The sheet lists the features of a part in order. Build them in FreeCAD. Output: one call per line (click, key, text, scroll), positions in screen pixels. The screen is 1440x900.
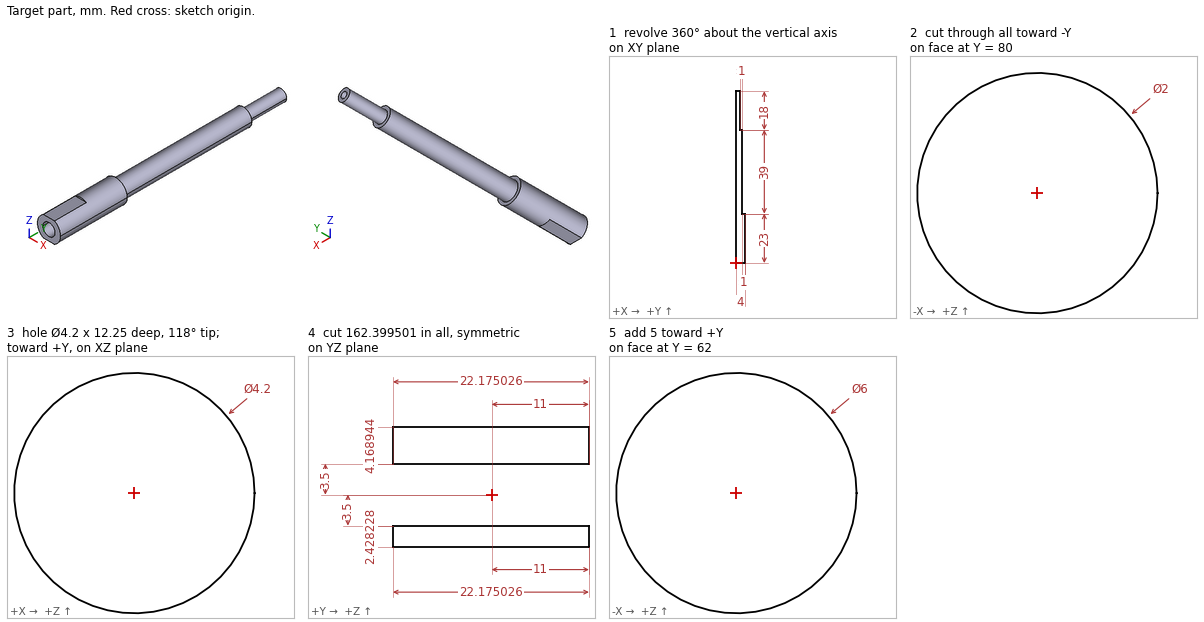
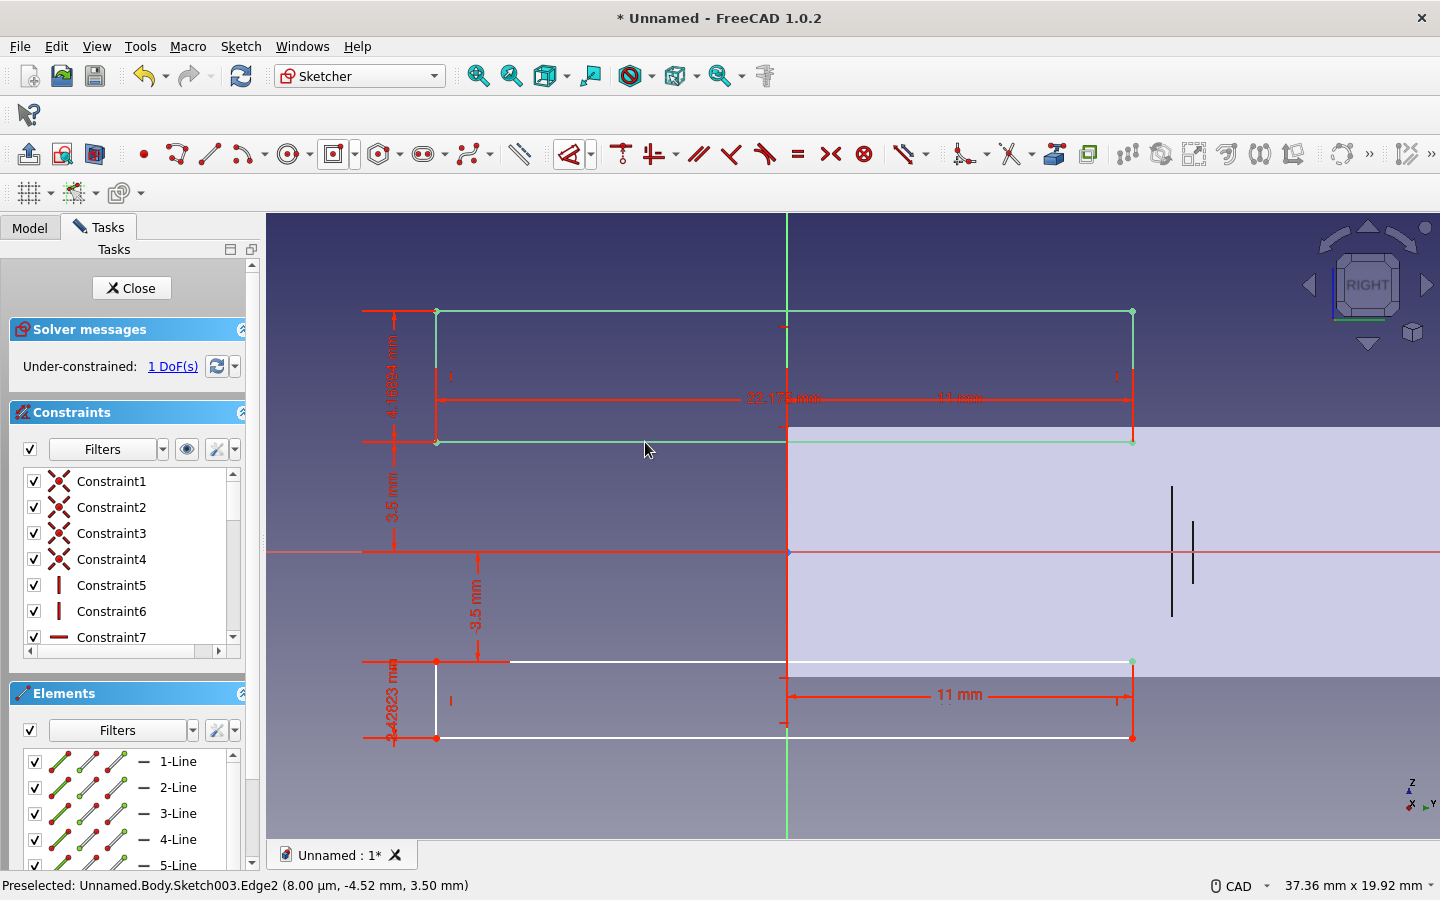
click(645, 738)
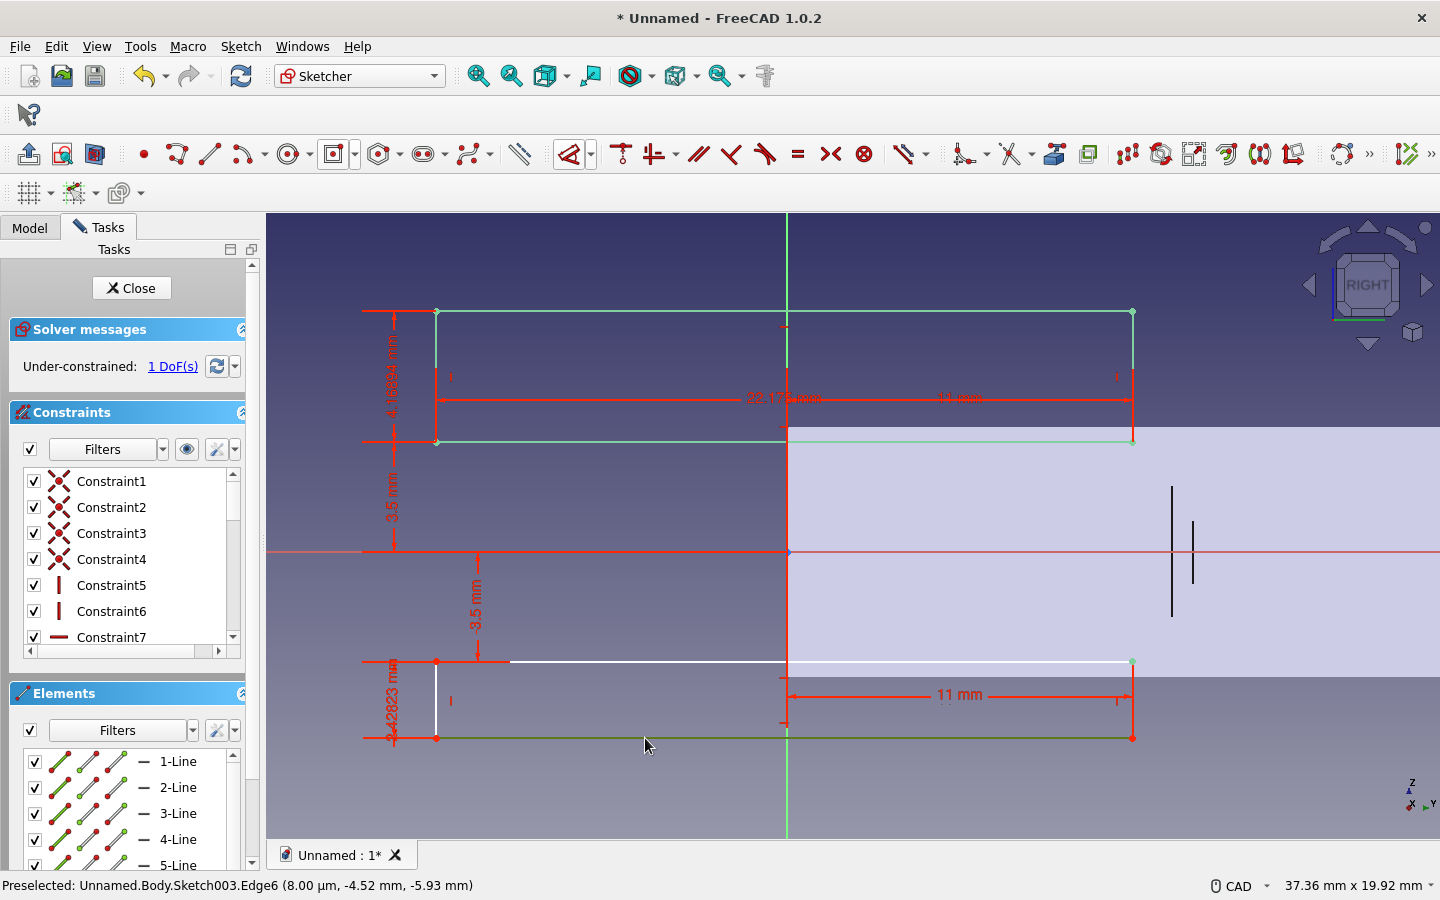
click(590, 154)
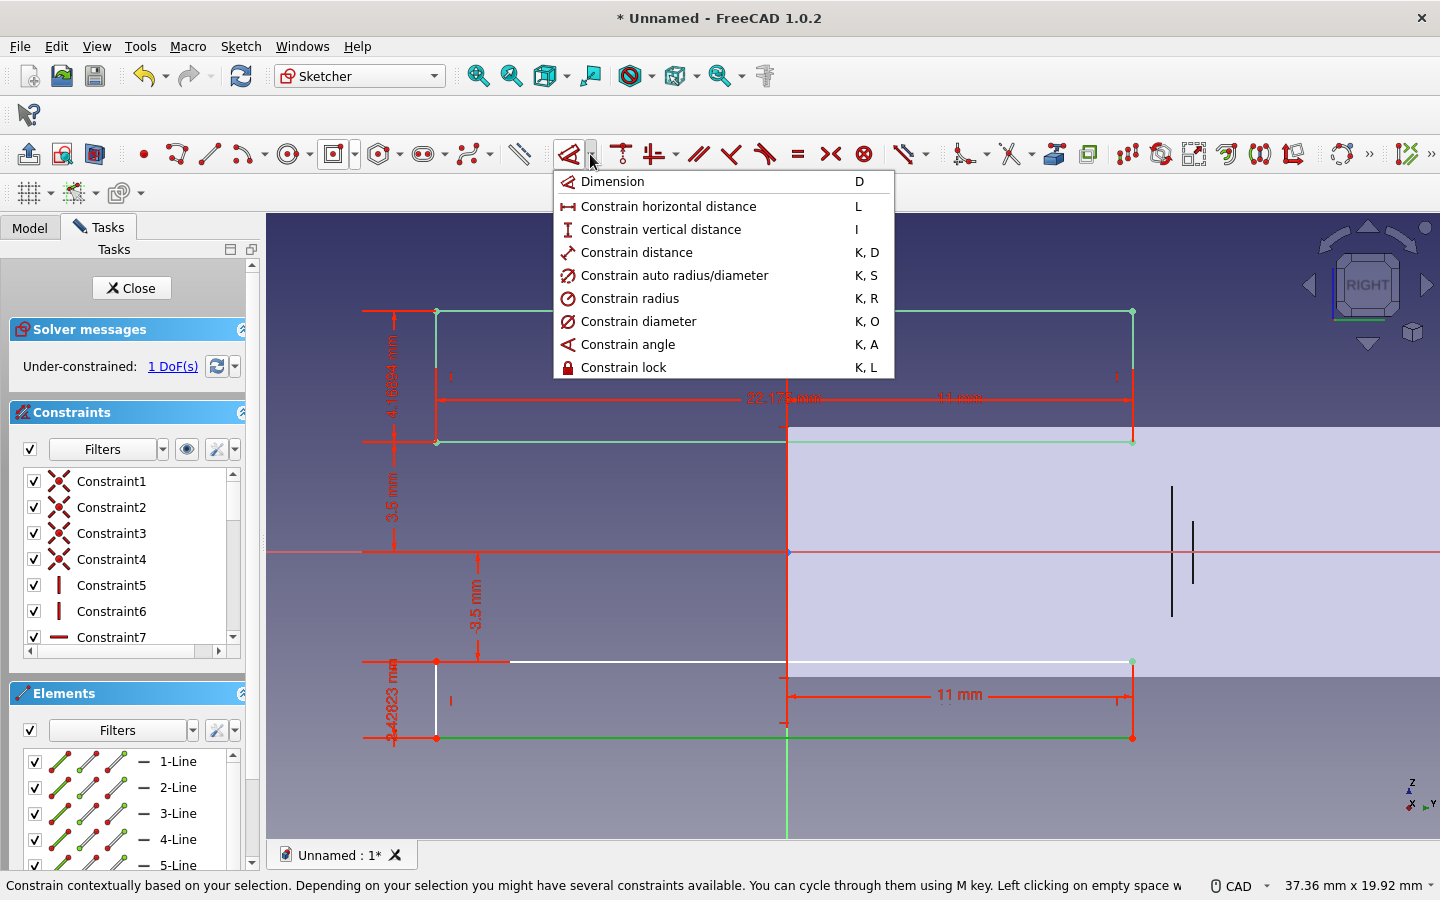
click(724, 206)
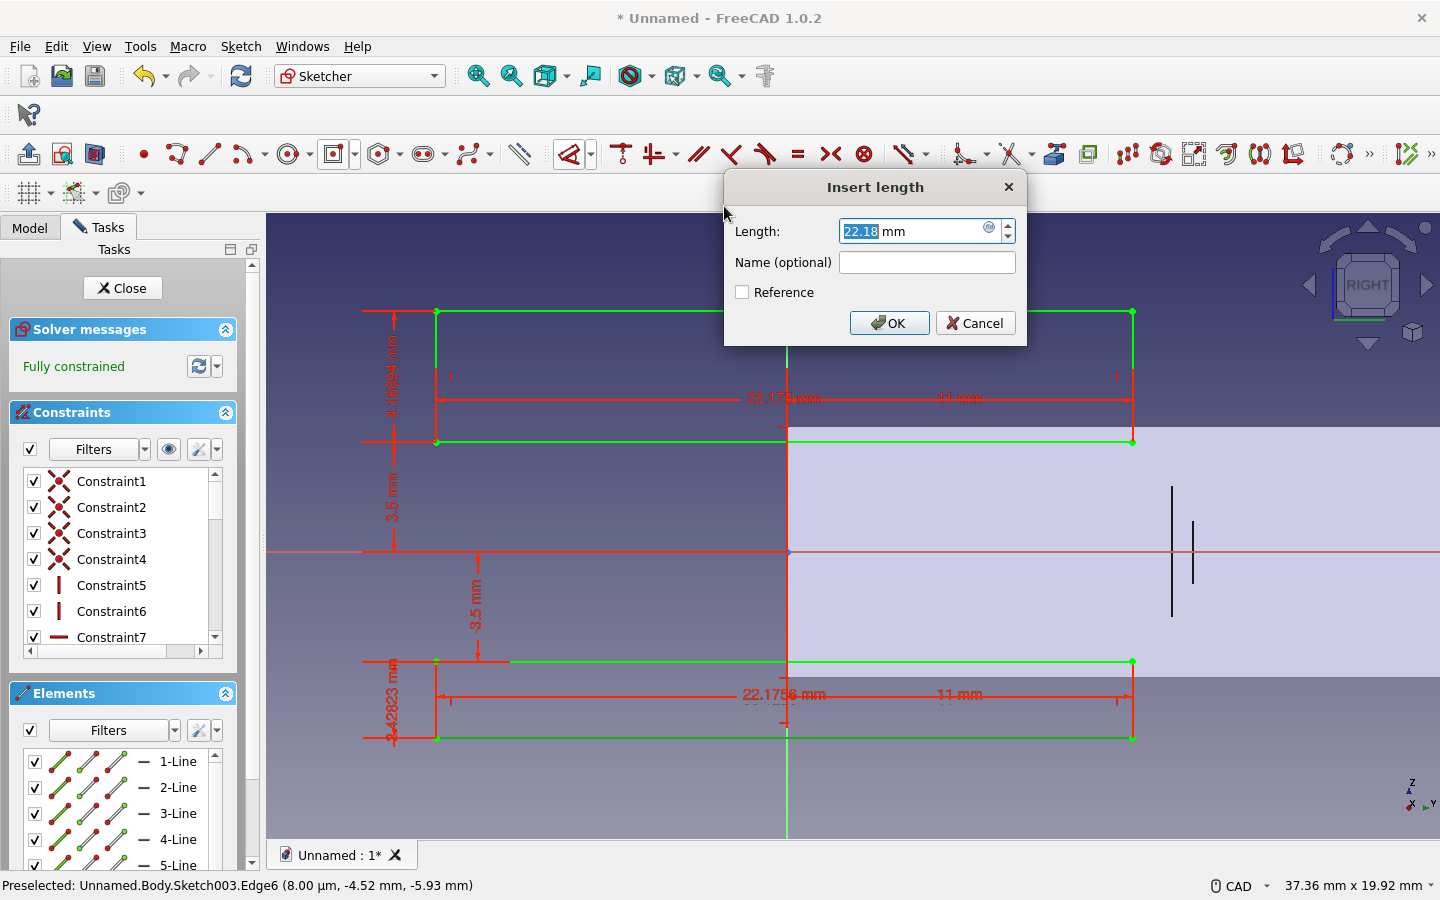
text(22.175026)
key(Return)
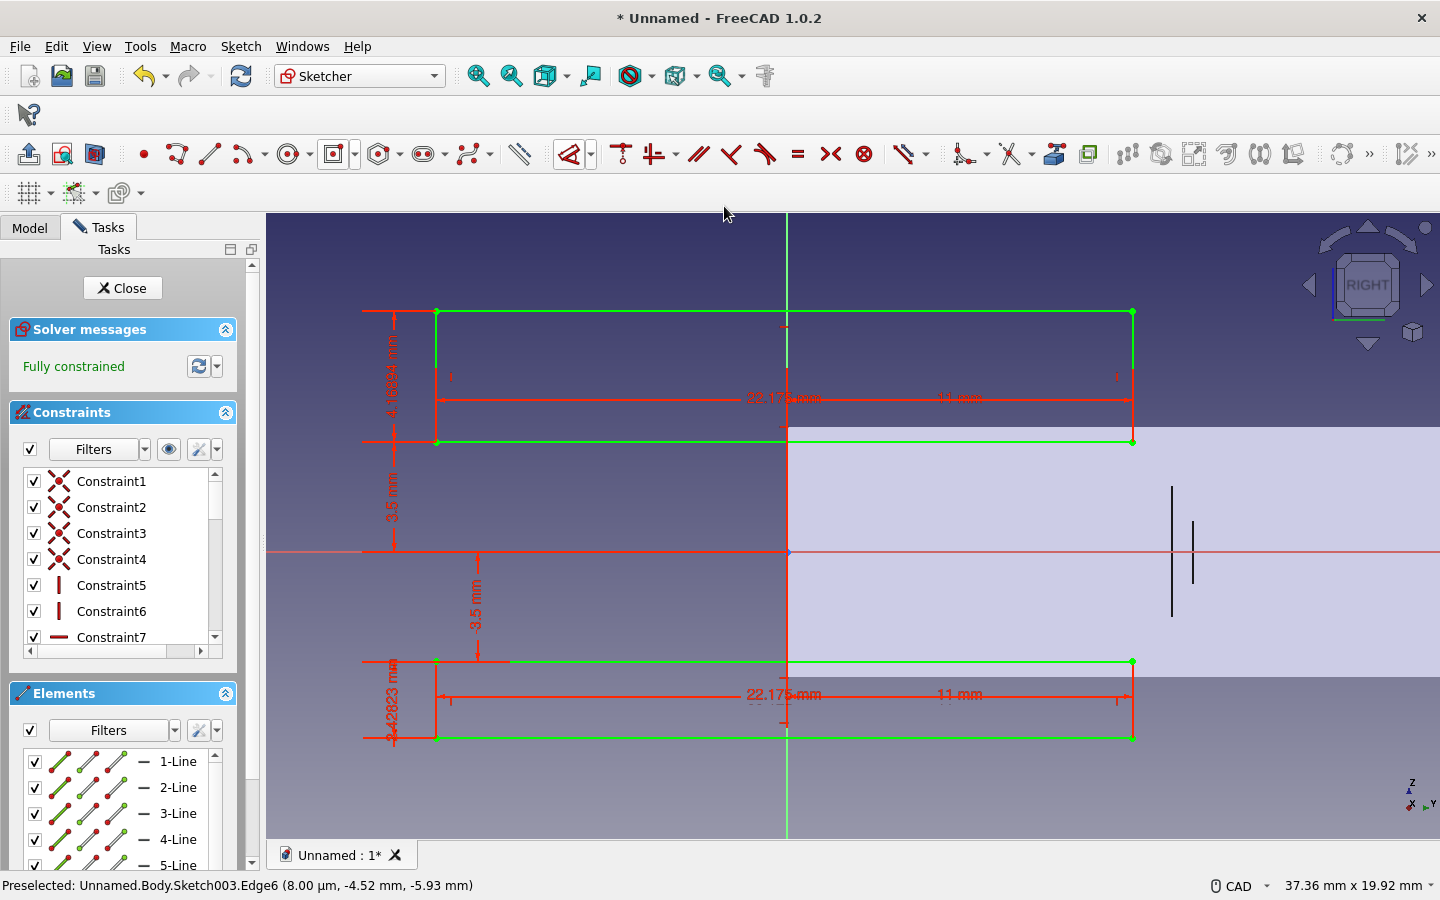
click(123, 288)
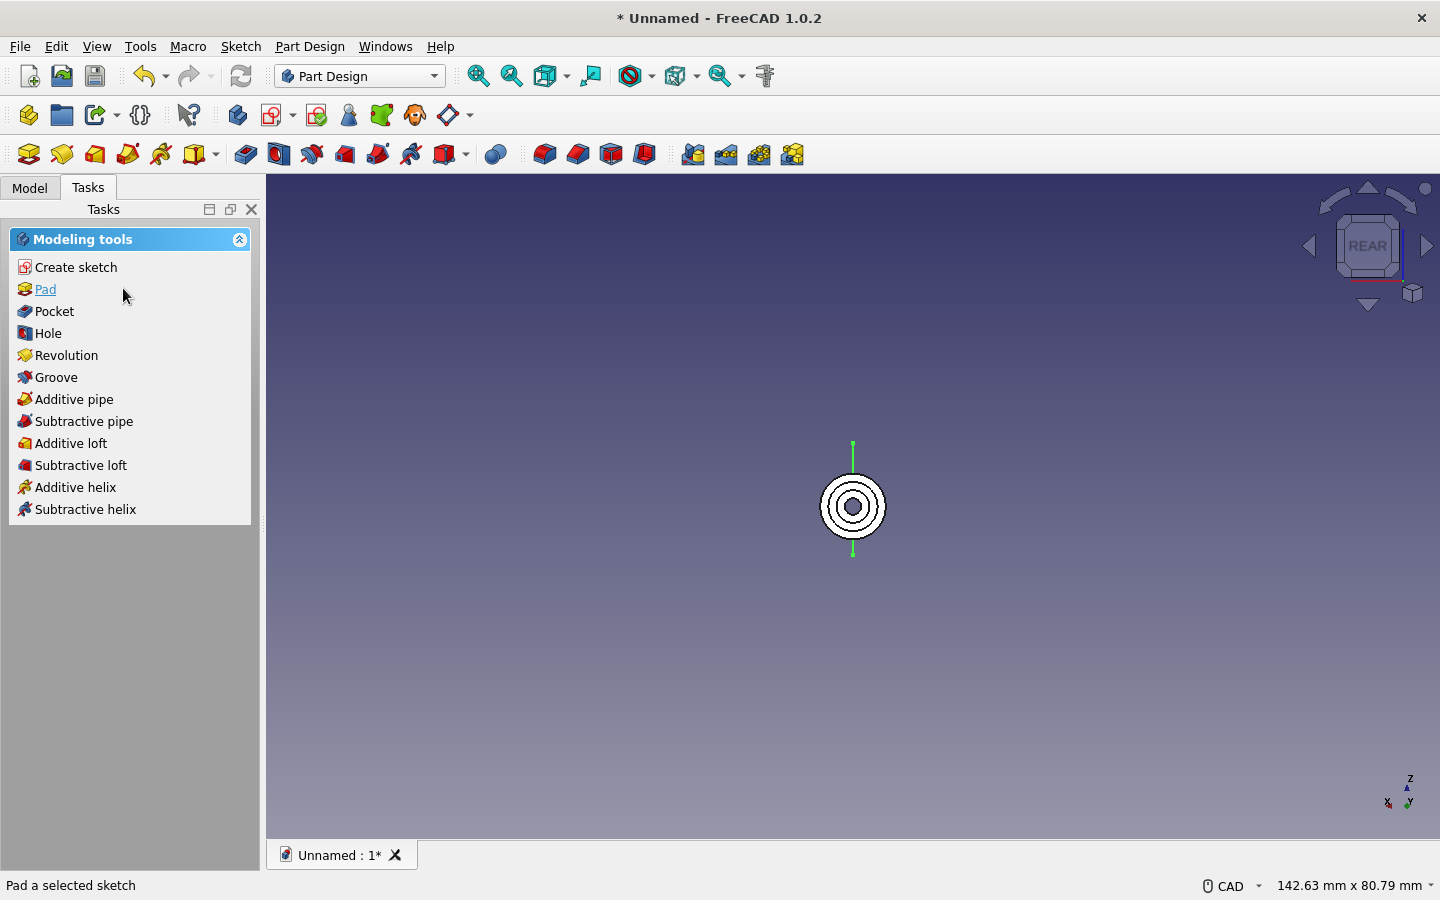
click(246, 154)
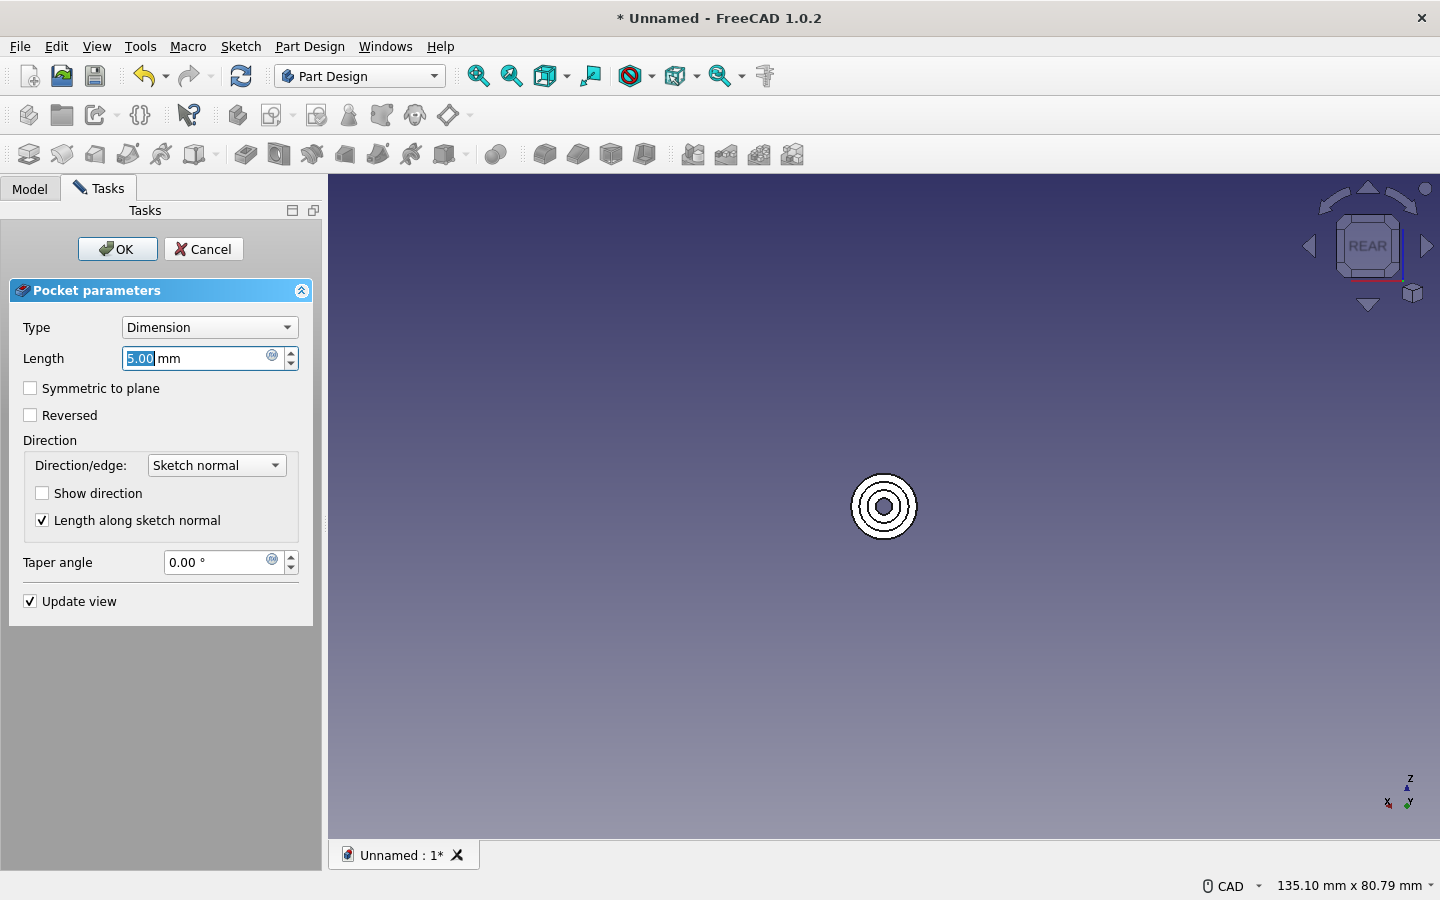
text(162.399501)
key(Tab)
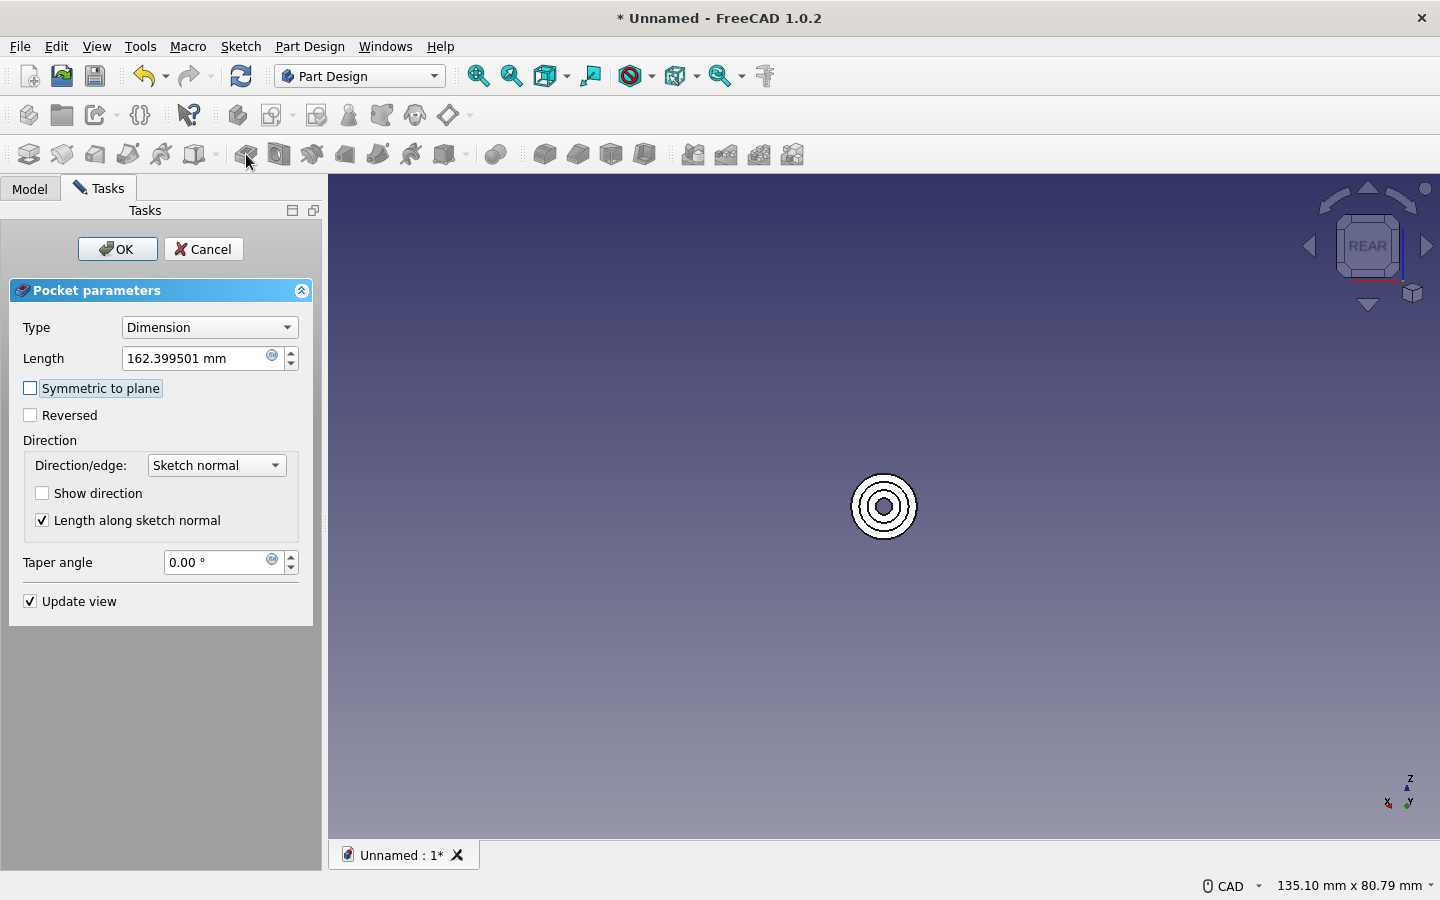
click(31, 388)